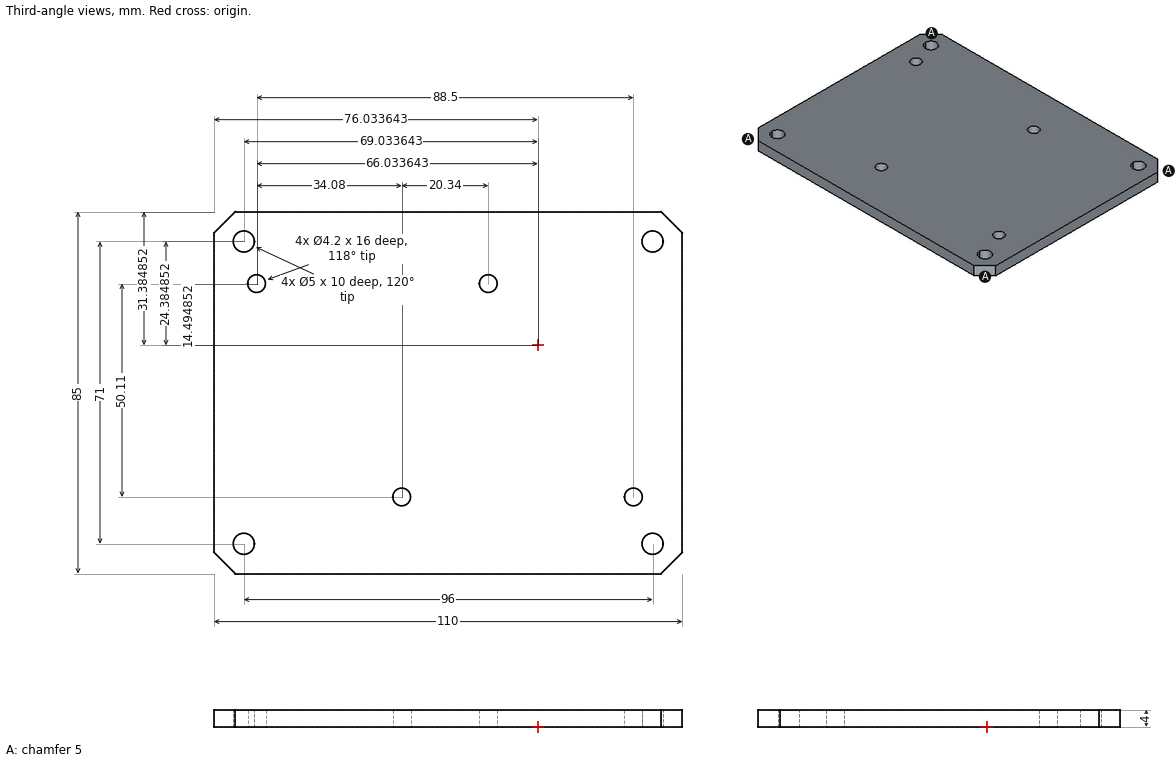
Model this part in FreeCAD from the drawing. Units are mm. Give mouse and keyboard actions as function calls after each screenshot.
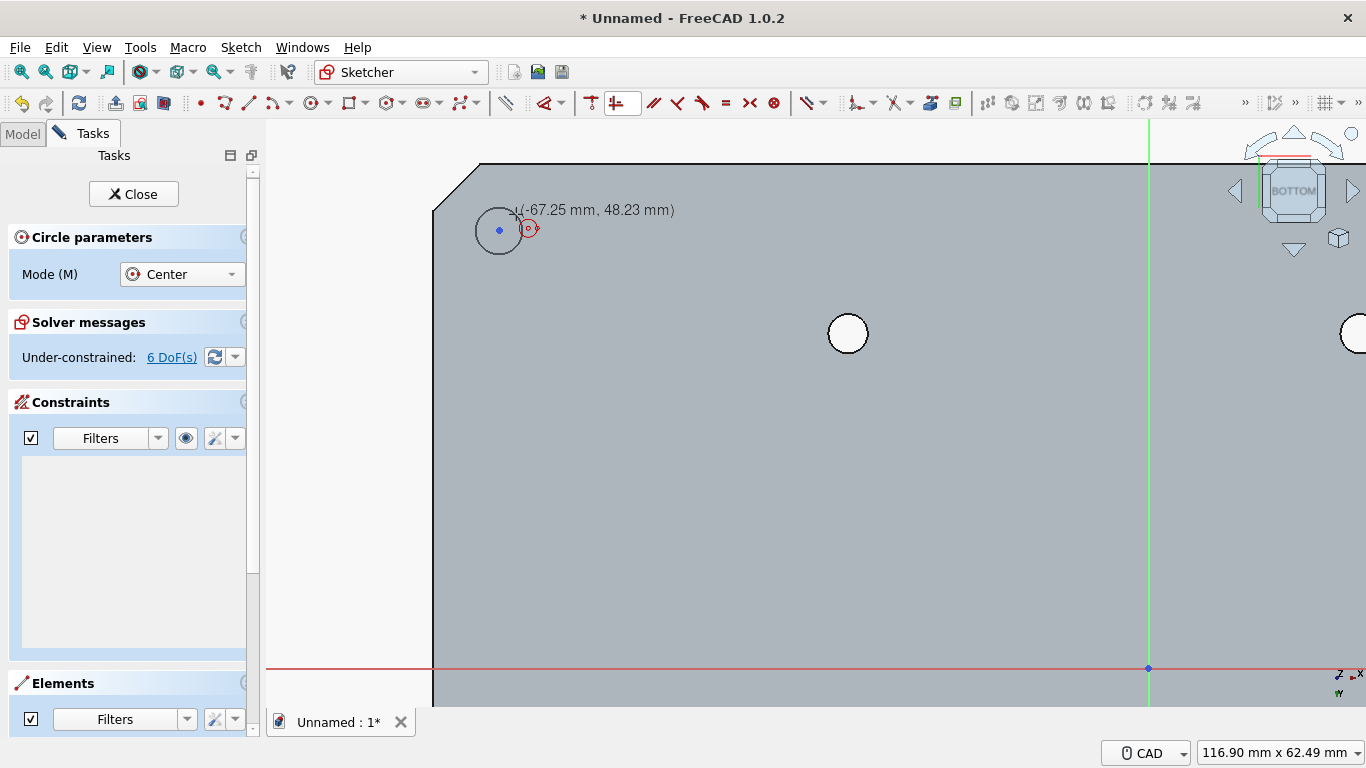
scroll(500, 229, down, 3)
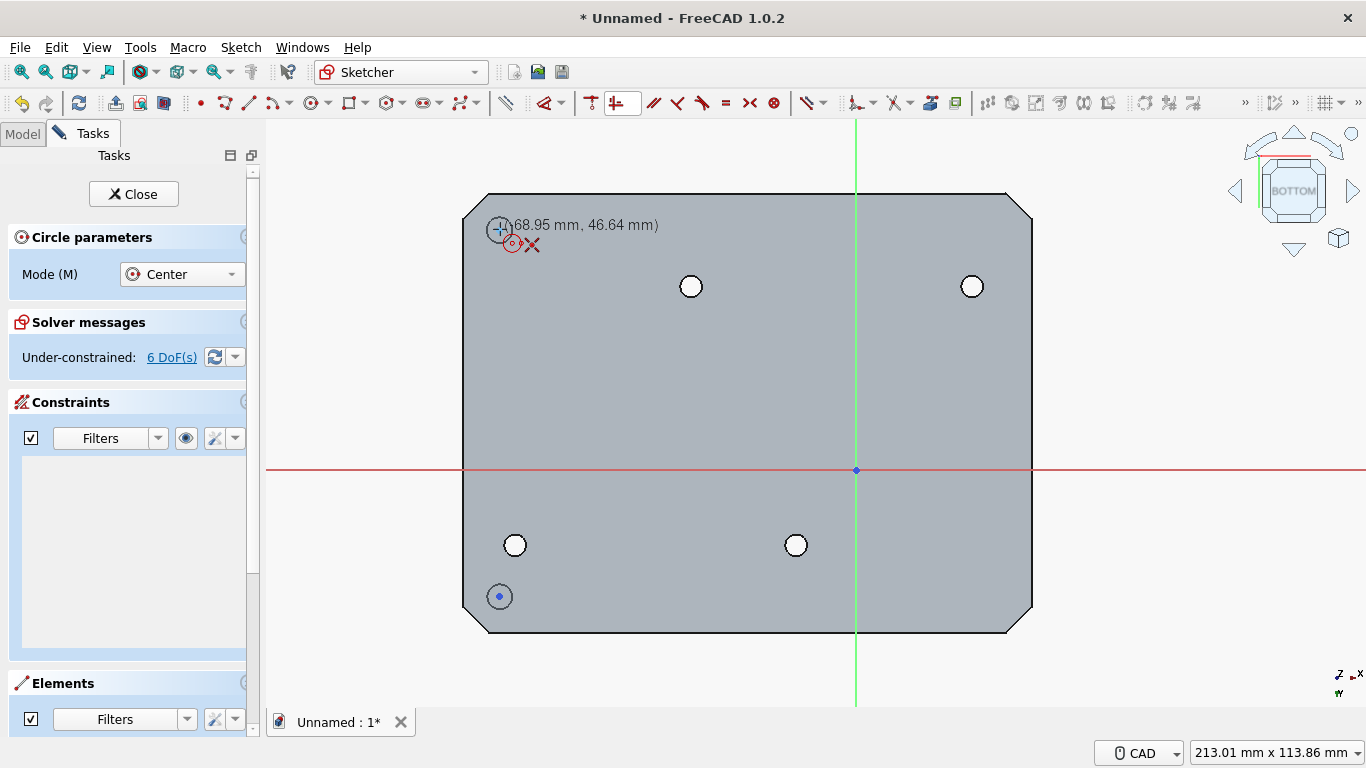
scroll(995, 230, up, 3)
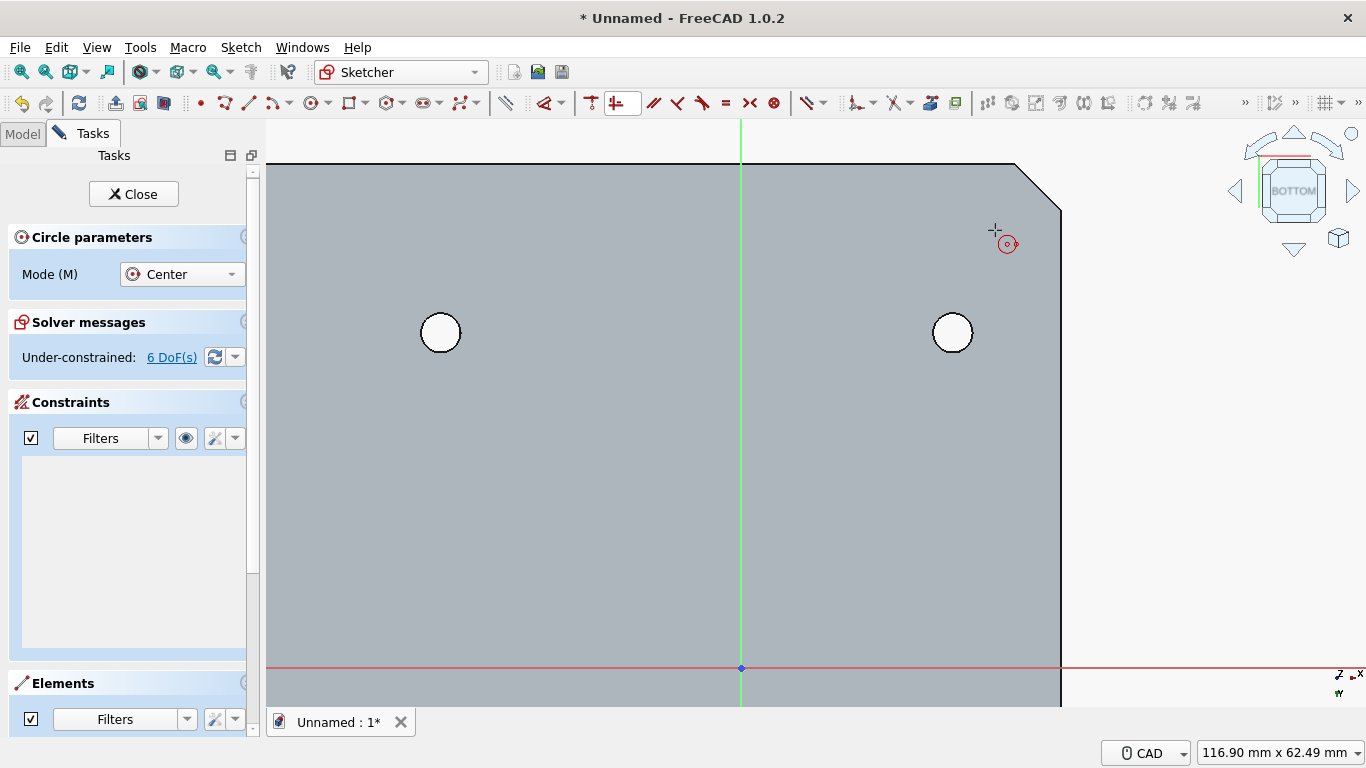
click(995, 229)
click(1012, 213)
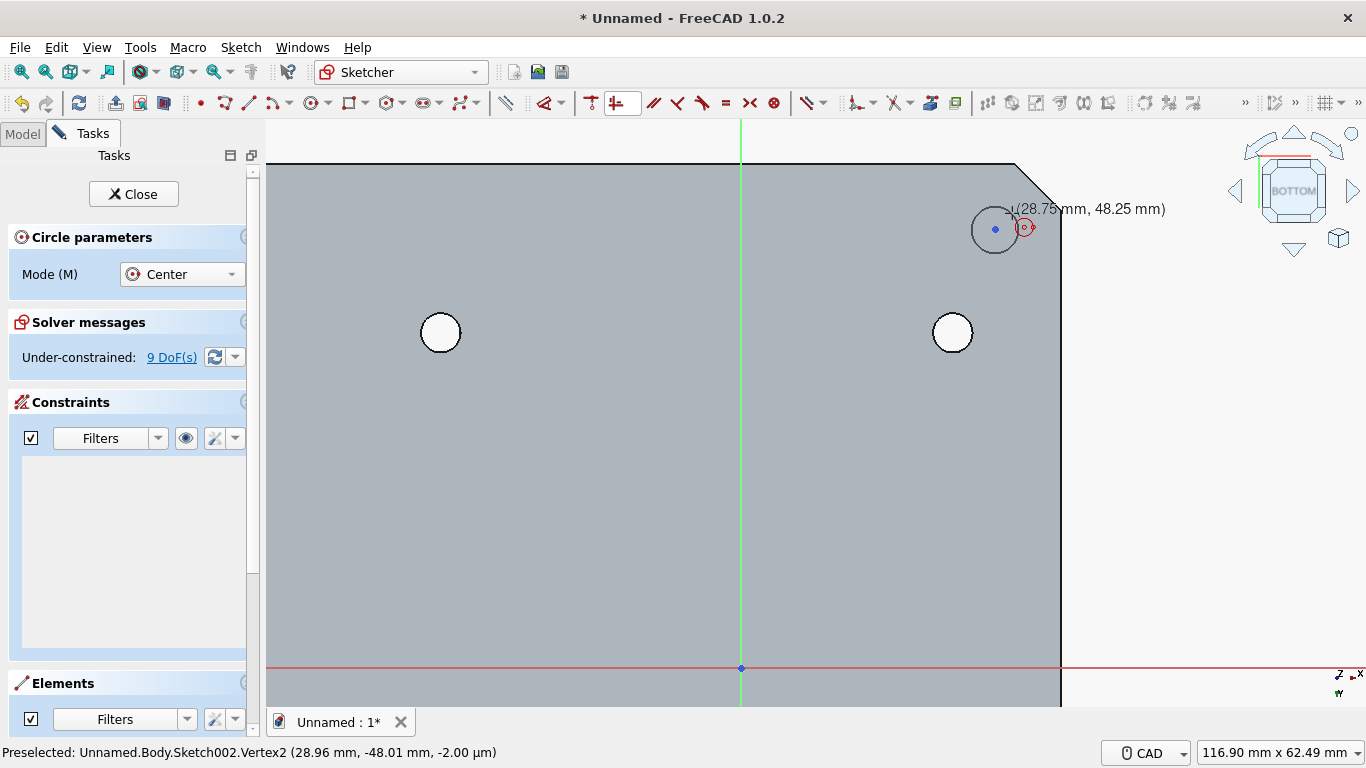
scroll(996, 230, down, 3)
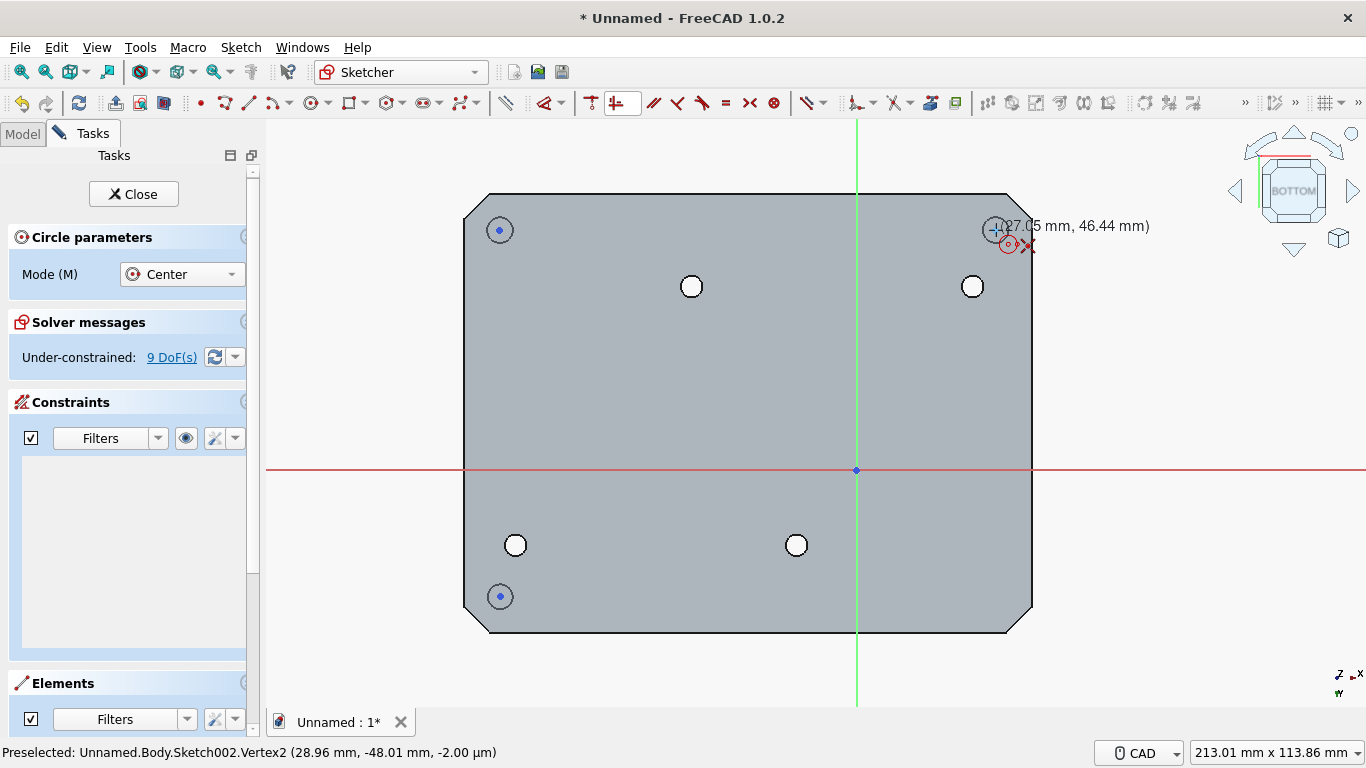
scroll(996, 596, up, 3)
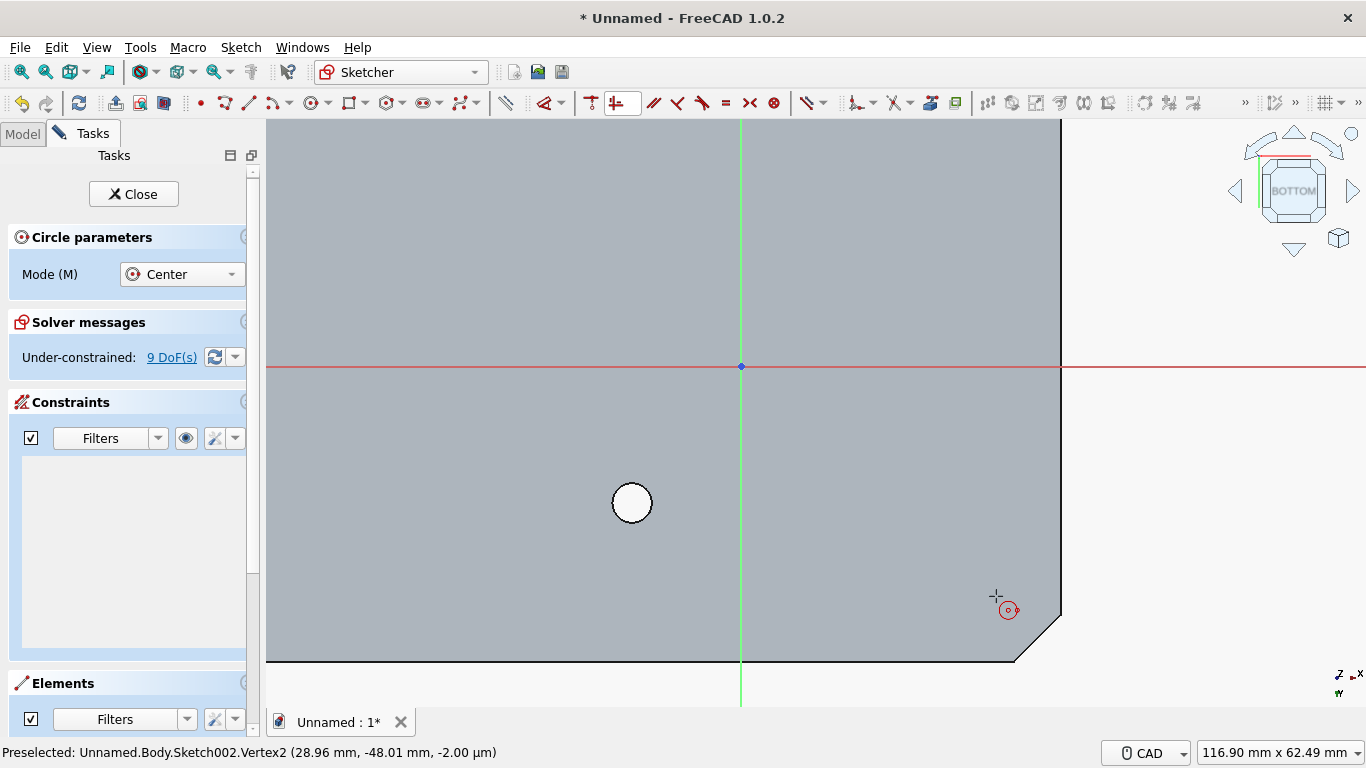
click(995, 596)
click(1012, 579)
key(Escape)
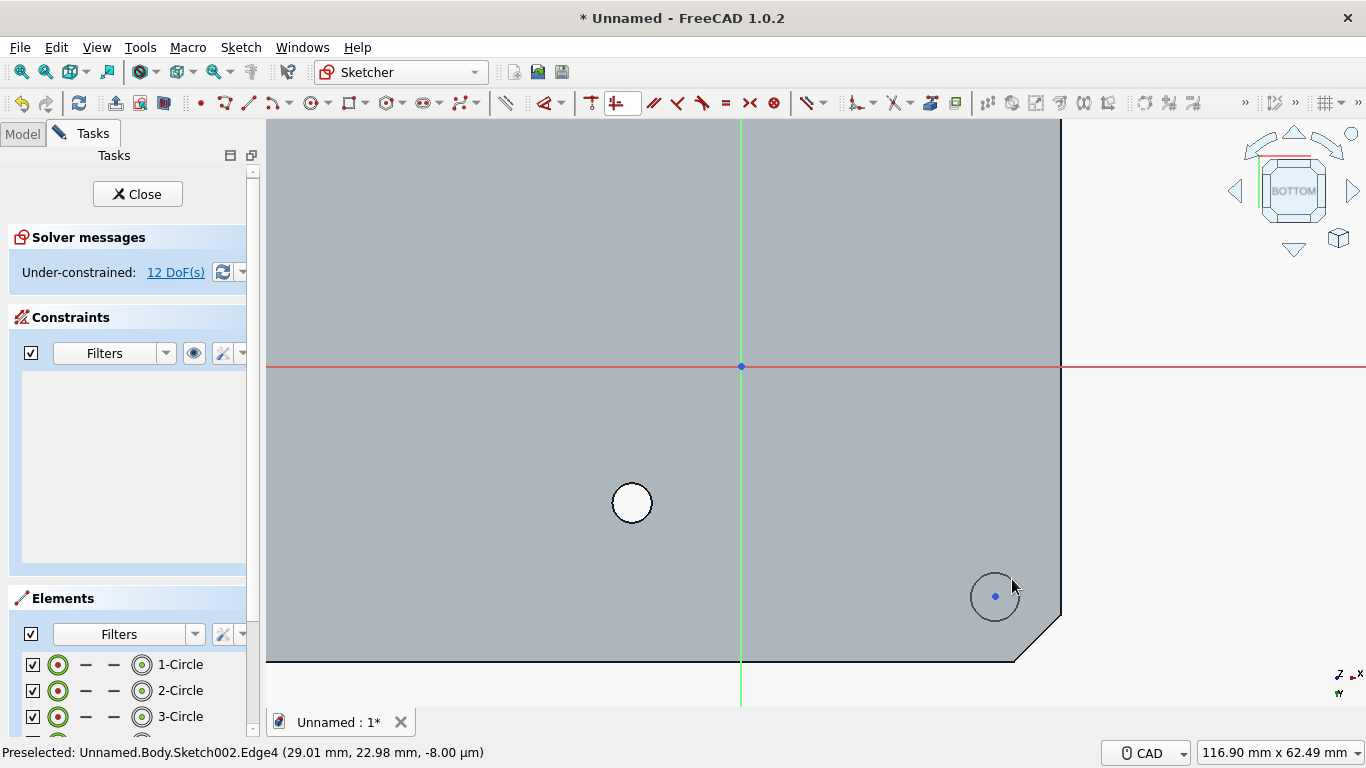
scroll(996, 597, down, 3)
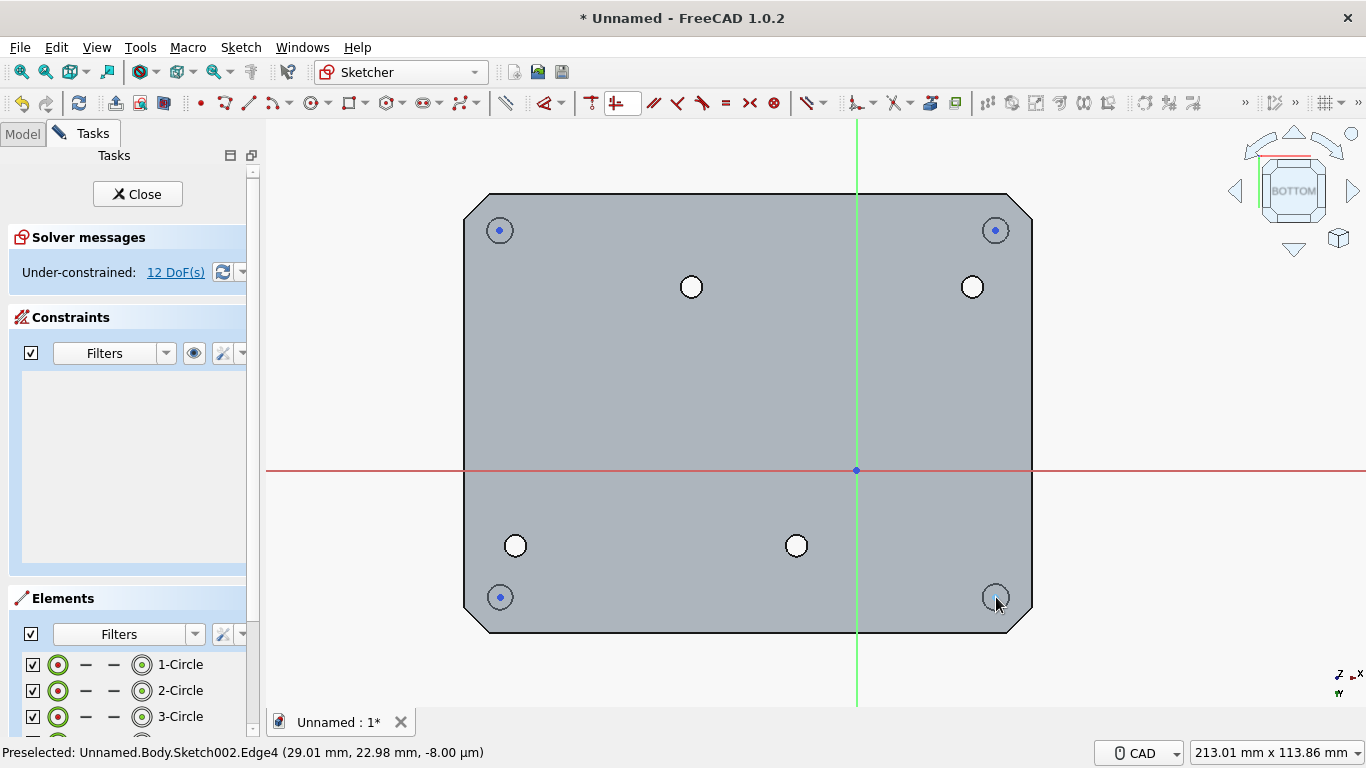
click(509, 588)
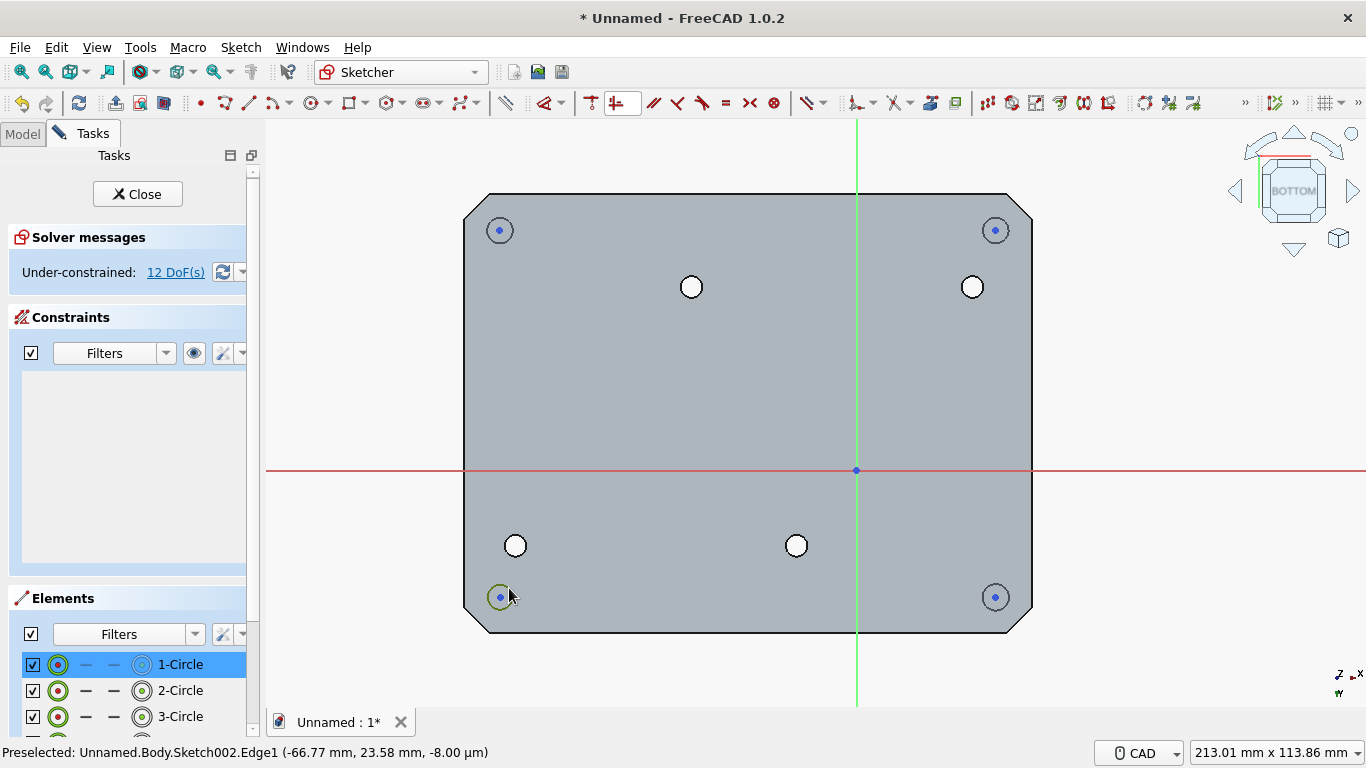
click(509, 222)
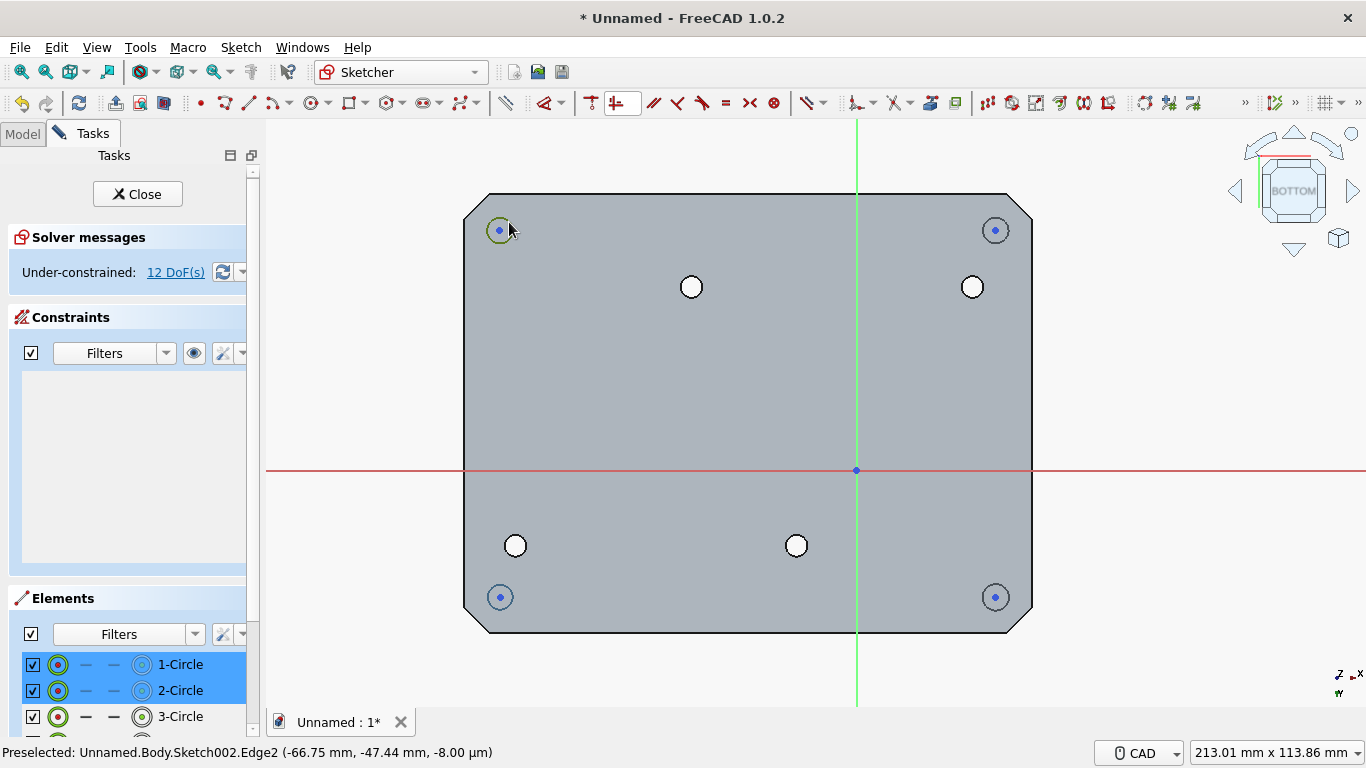
click(1005, 221)